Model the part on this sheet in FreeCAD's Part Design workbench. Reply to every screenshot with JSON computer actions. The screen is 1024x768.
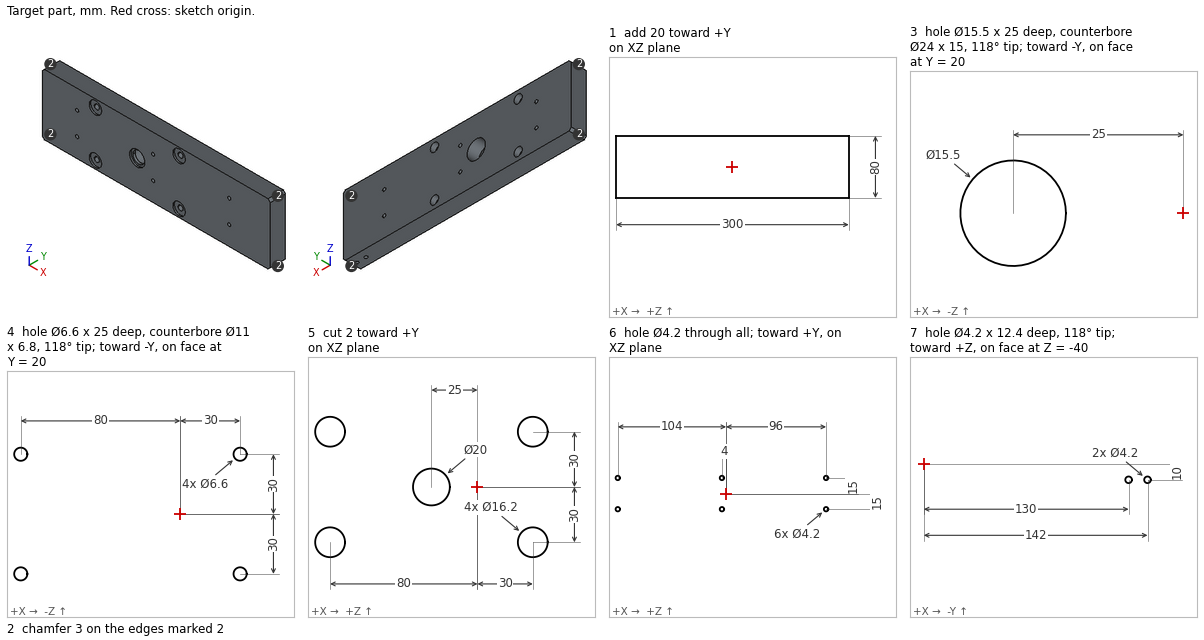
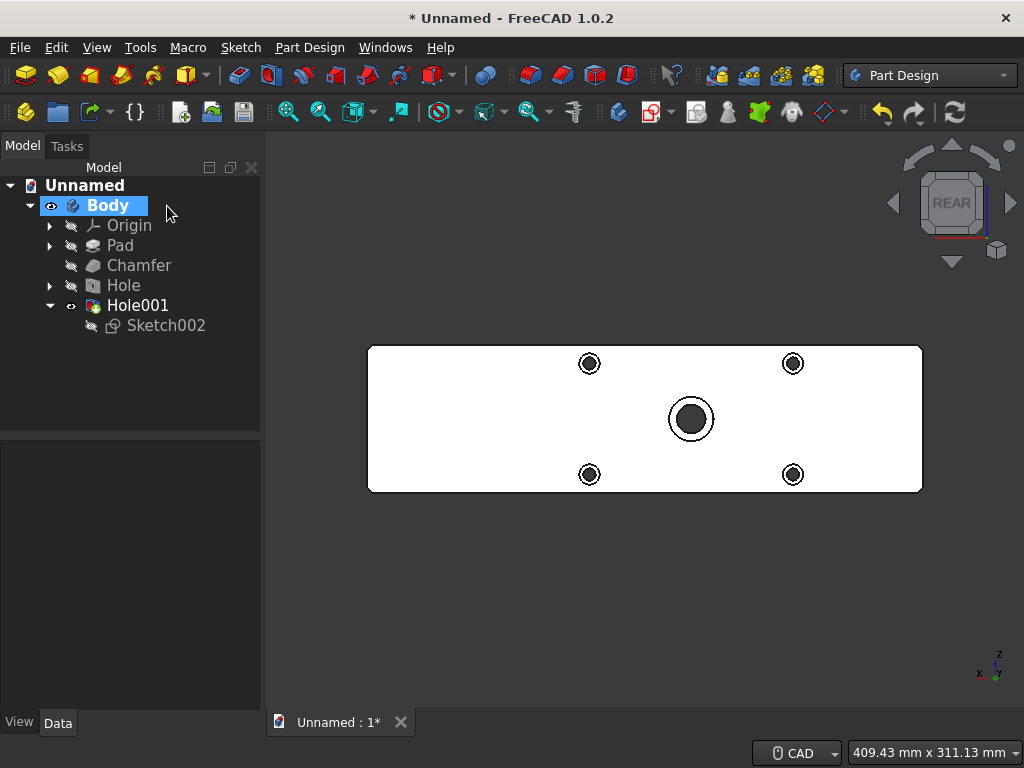
{"action": "left_click", "coordinate": [652, 112]}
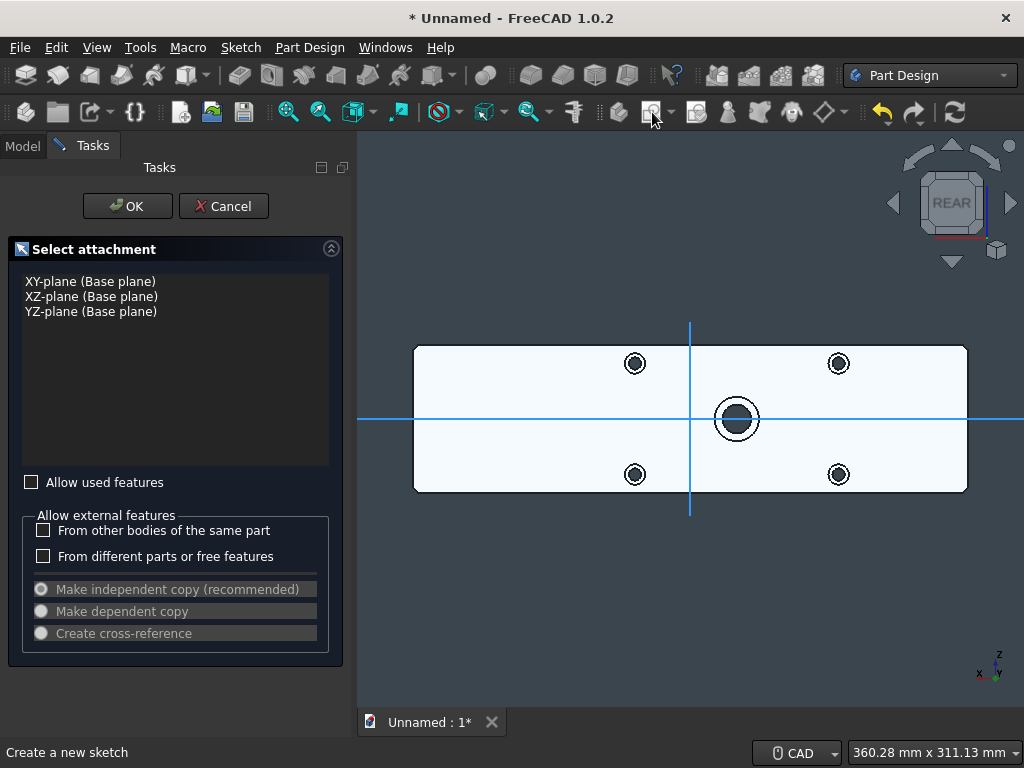
{"action": "left_click", "coordinate": [82, 296]}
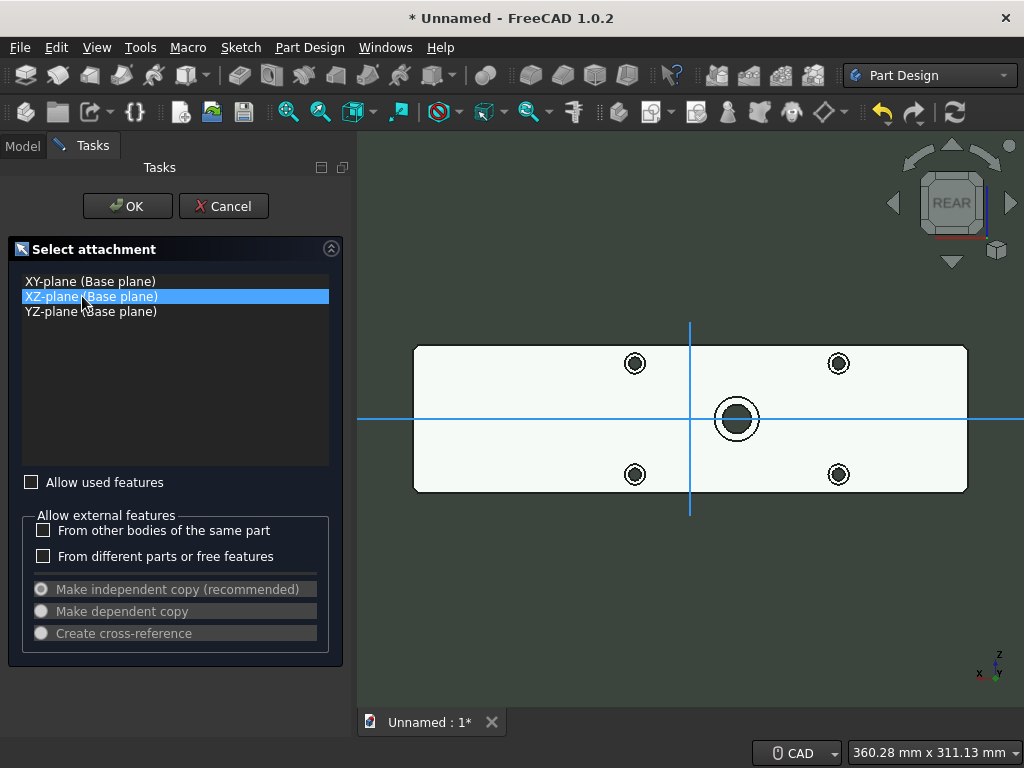
{"action": "left_click", "coordinate": [128, 206]}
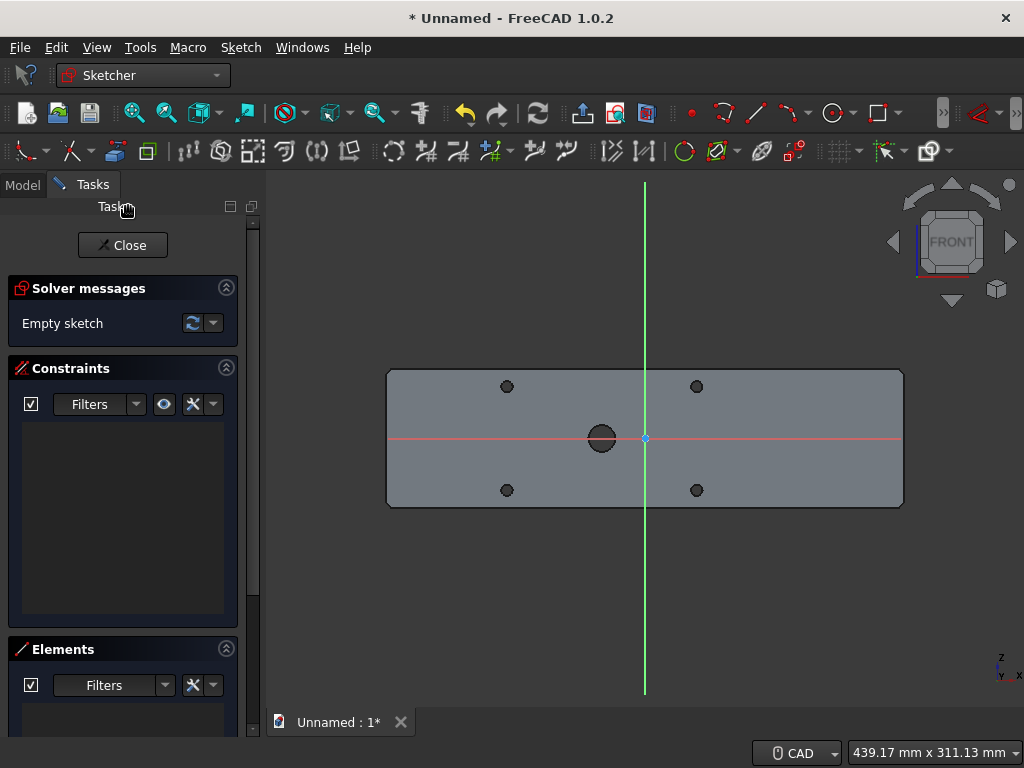
{"action": "scroll", "coordinate": [633, 439], "scroll_direction": "up", "scroll_amount": 3}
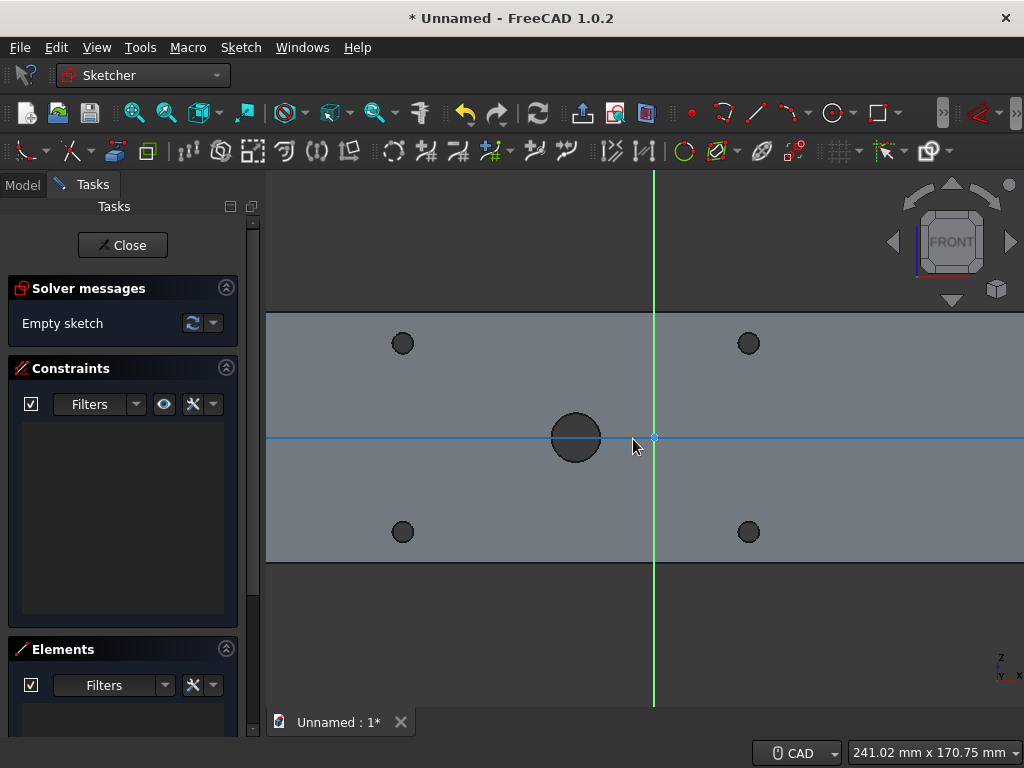
{"action": "left_click", "coordinate": [834, 114]}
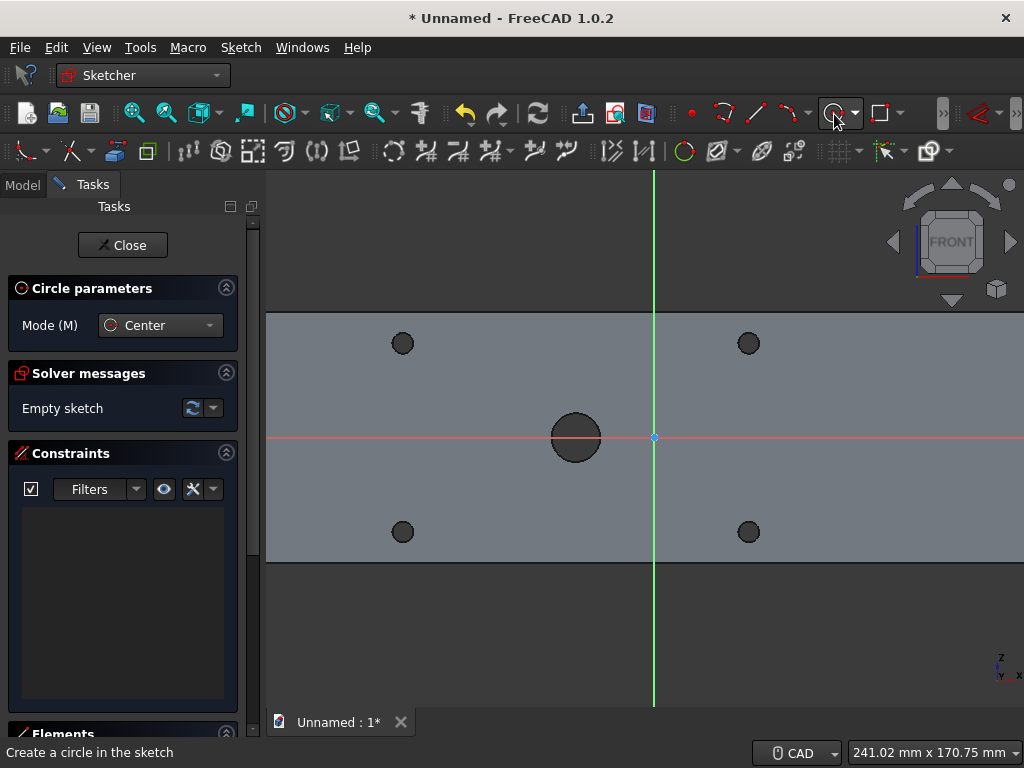
{"action": "left_click", "coordinate": [576, 438]}
{"action": "mouse_move", "coordinate": [598, 415]}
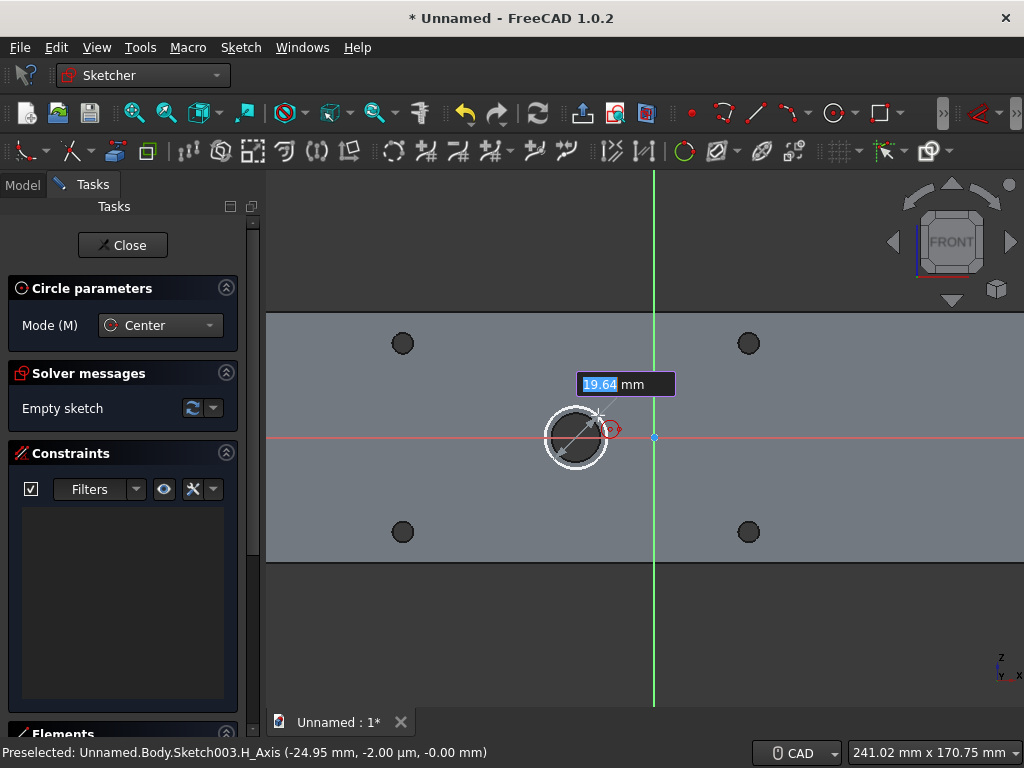
{"action": "type", "text": "20"}
{"action": "key", "text": "Return"}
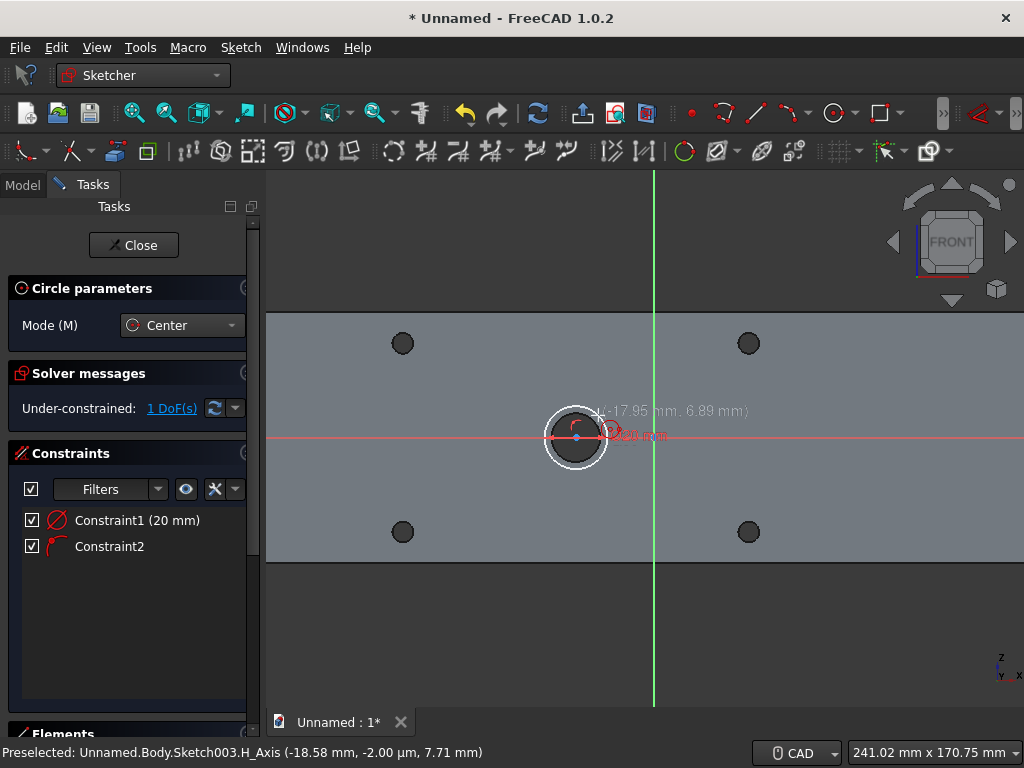
{"action": "left_click", "coordinate": [749, 532]}
{"action": "mouse_move", "coordinate": [767, 514]}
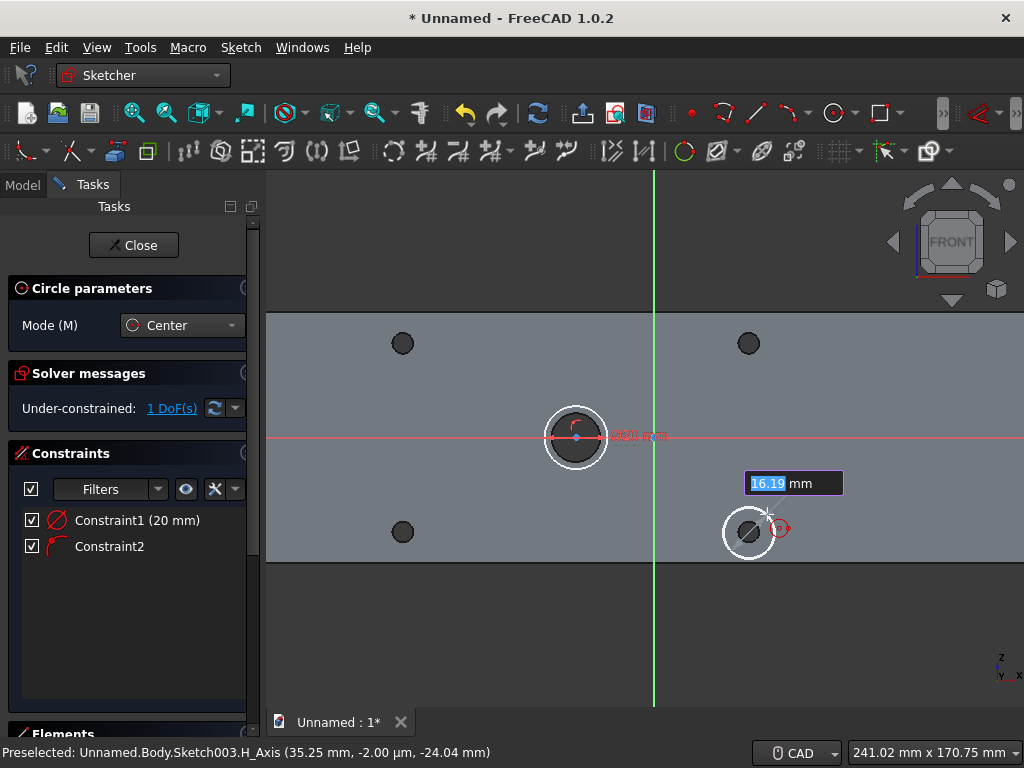
{"action": "type", "text": "16.2"}
{"action": "key", "text": "Return"}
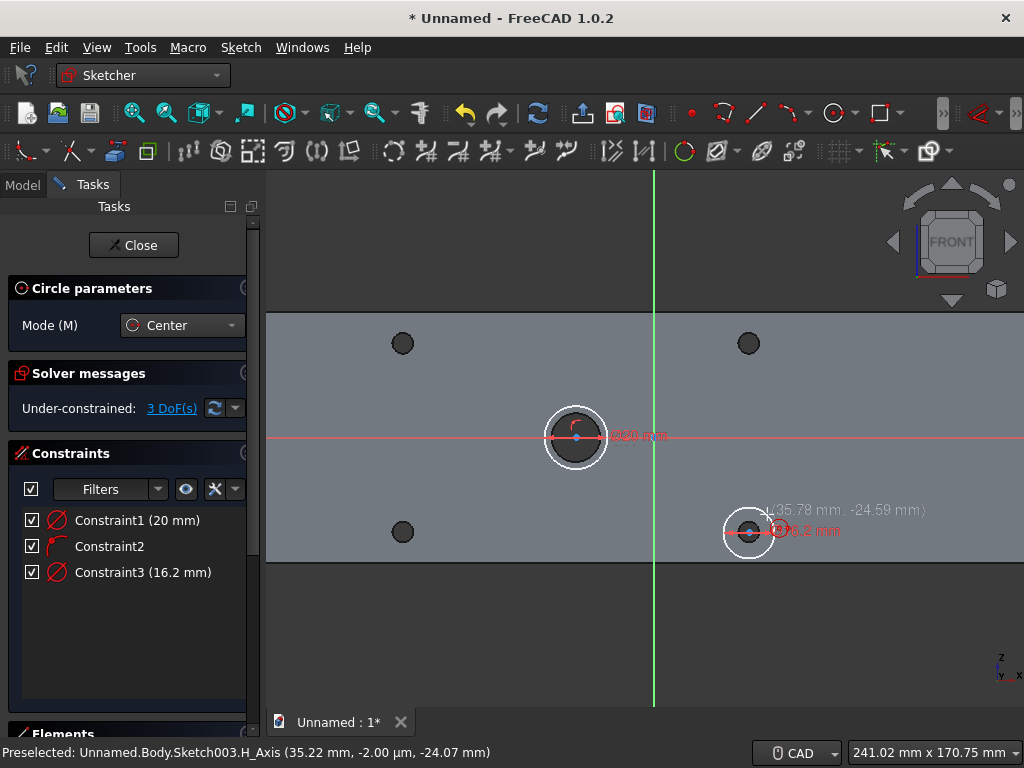
{"action": "left_click", "coordinate": [403, 532]}
{"action": "mouse_move", "coordinate": [421, 514]}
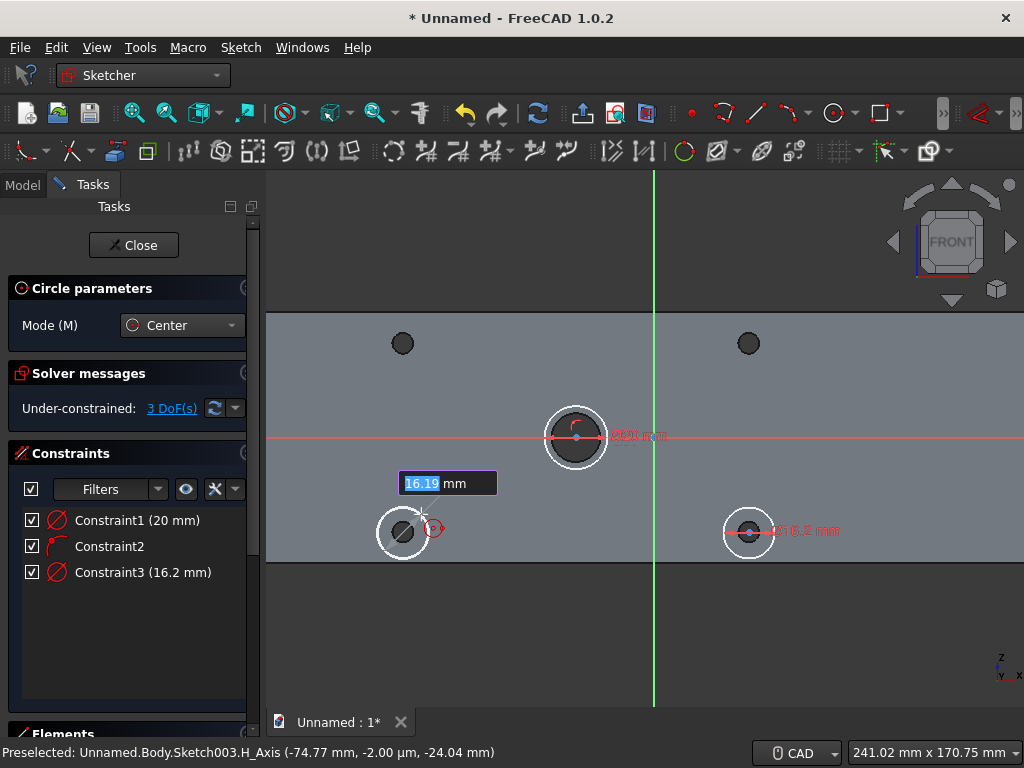
{"action": "type", "text": "16.2"}
{"action": "key", "text": "Return"}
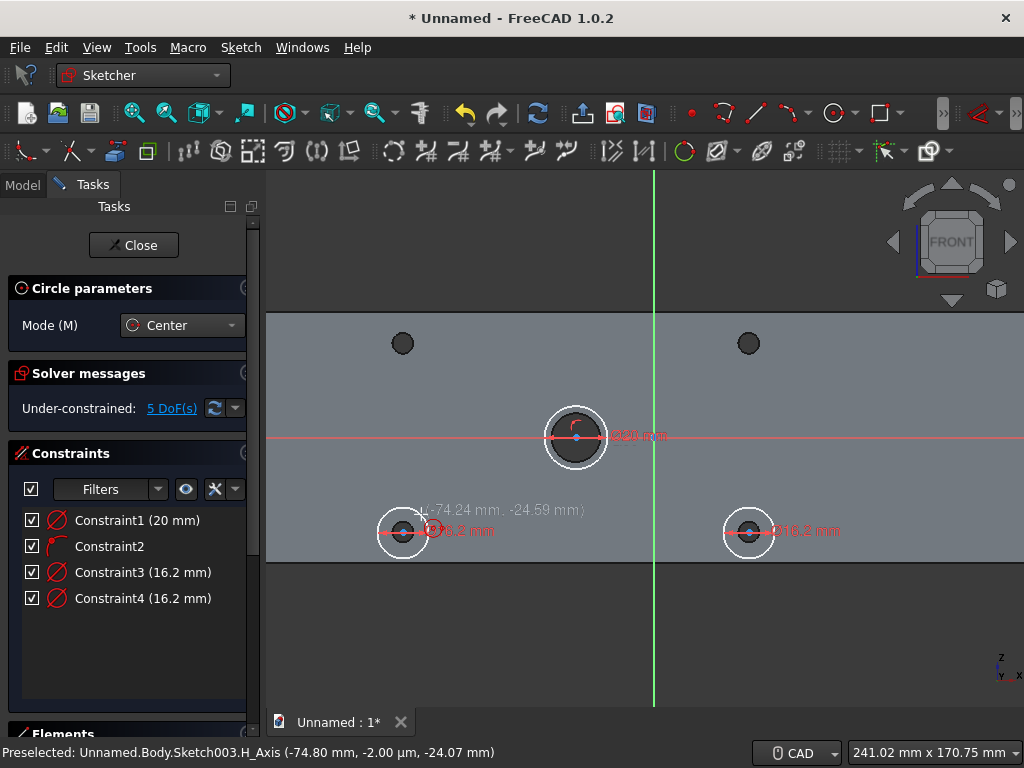
{"action": "left_click", "coordinate": [749, 343]}
{"action": "mouse_move", "coordinate": [767, 325]}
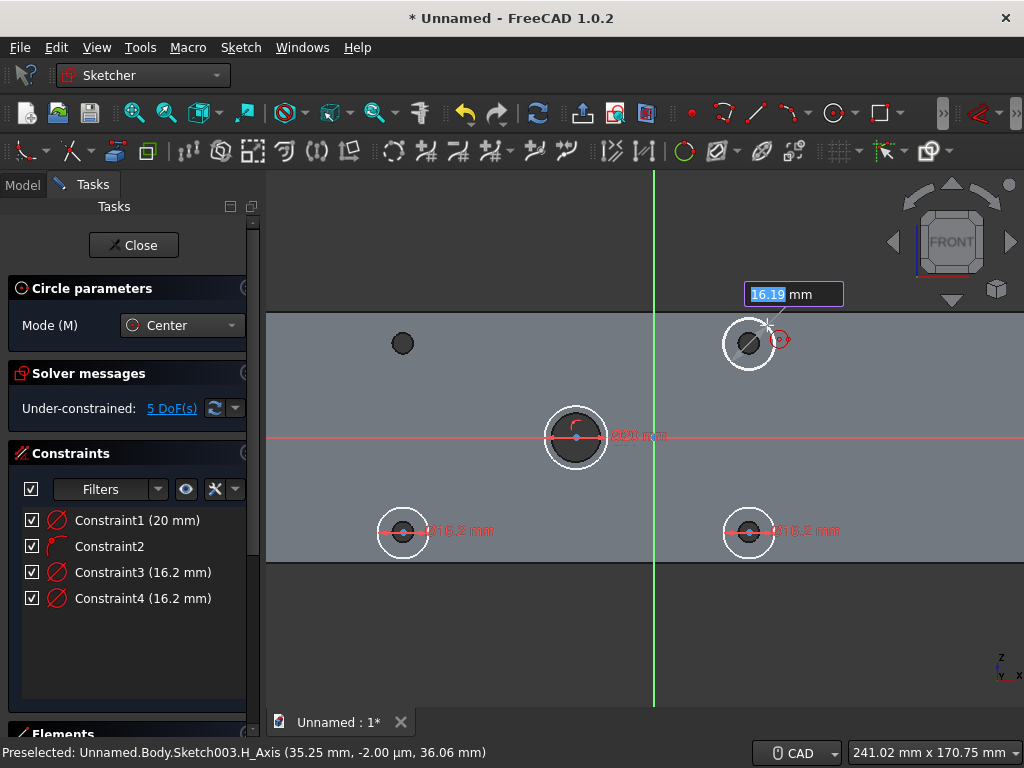
{"action": "type", "text": "16.2"}
{"action": "key", "text": "Return"}